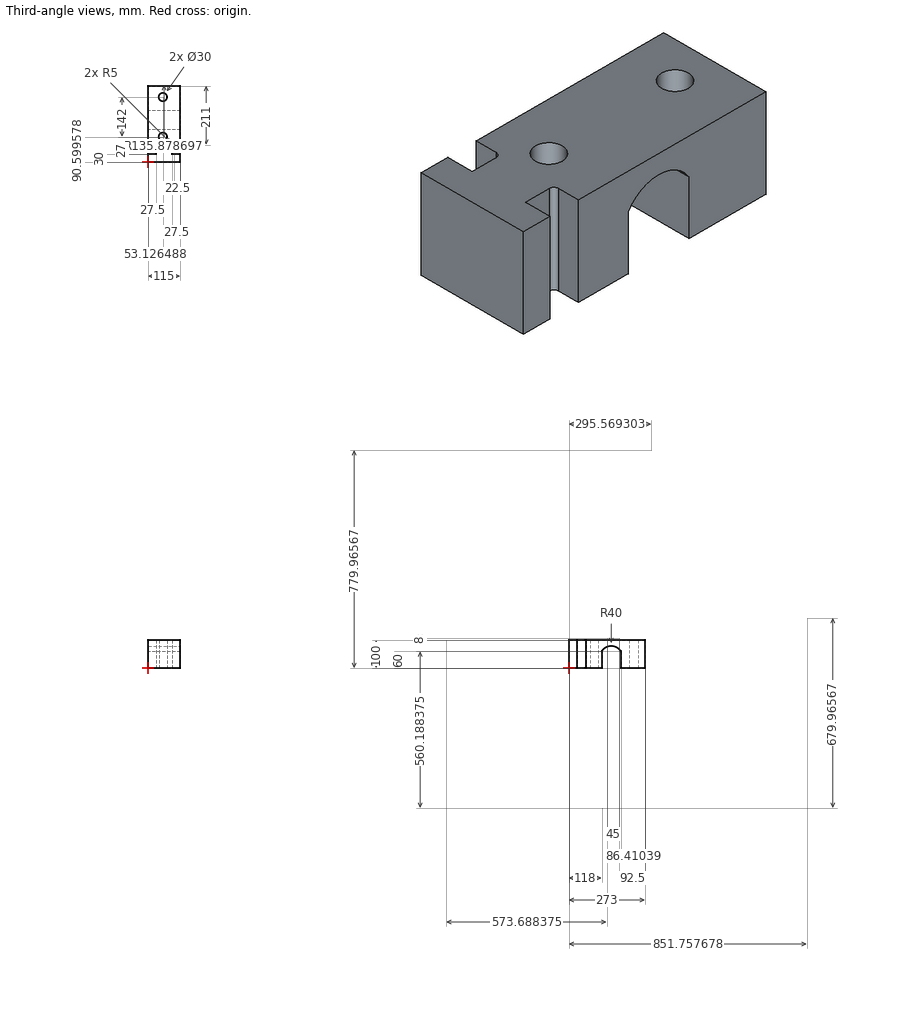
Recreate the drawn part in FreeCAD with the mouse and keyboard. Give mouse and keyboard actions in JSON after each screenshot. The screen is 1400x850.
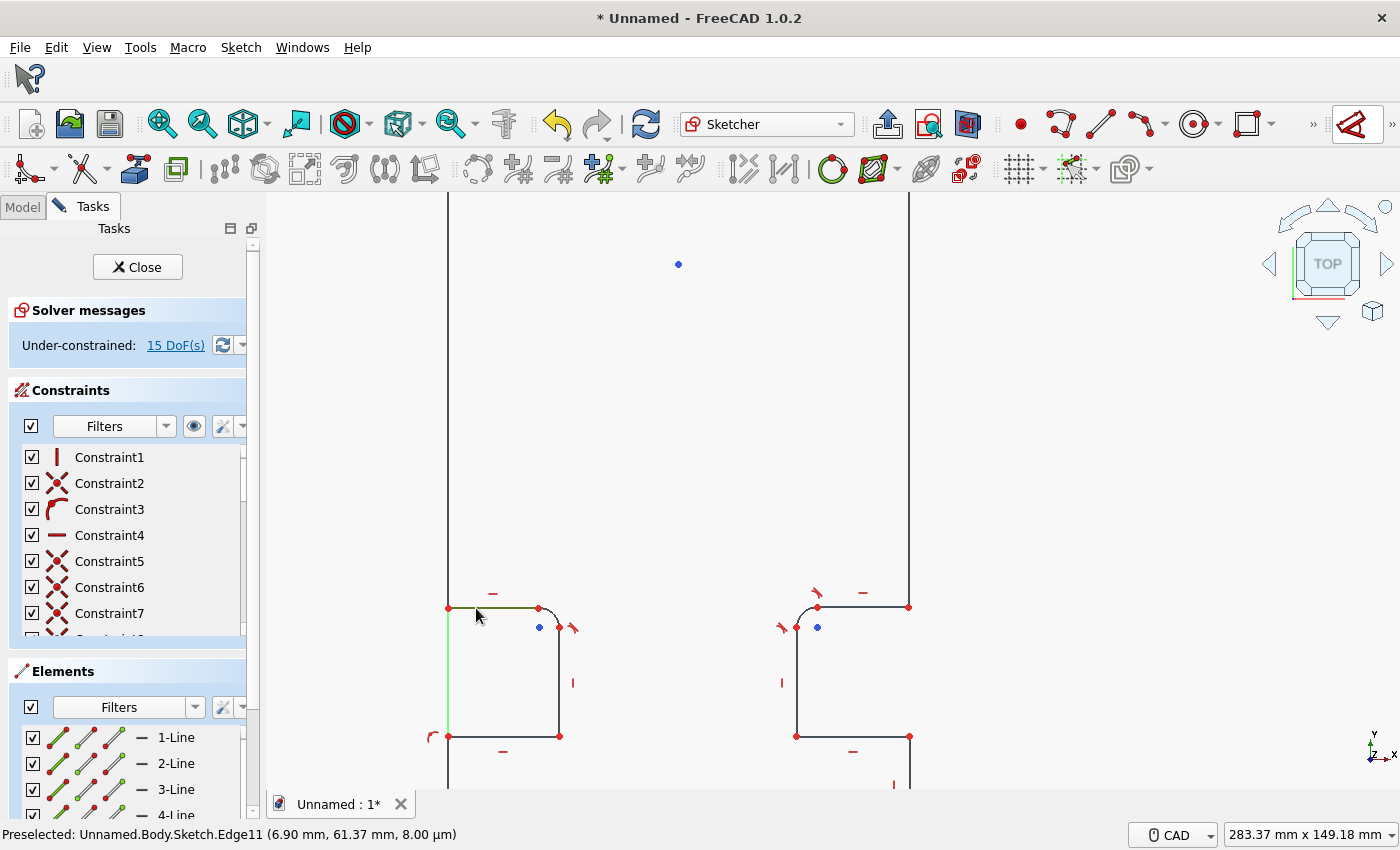
{"action": "scroll", "coordinate": [557, 619], "scroll_direction": "up", "scroll_amount": 2}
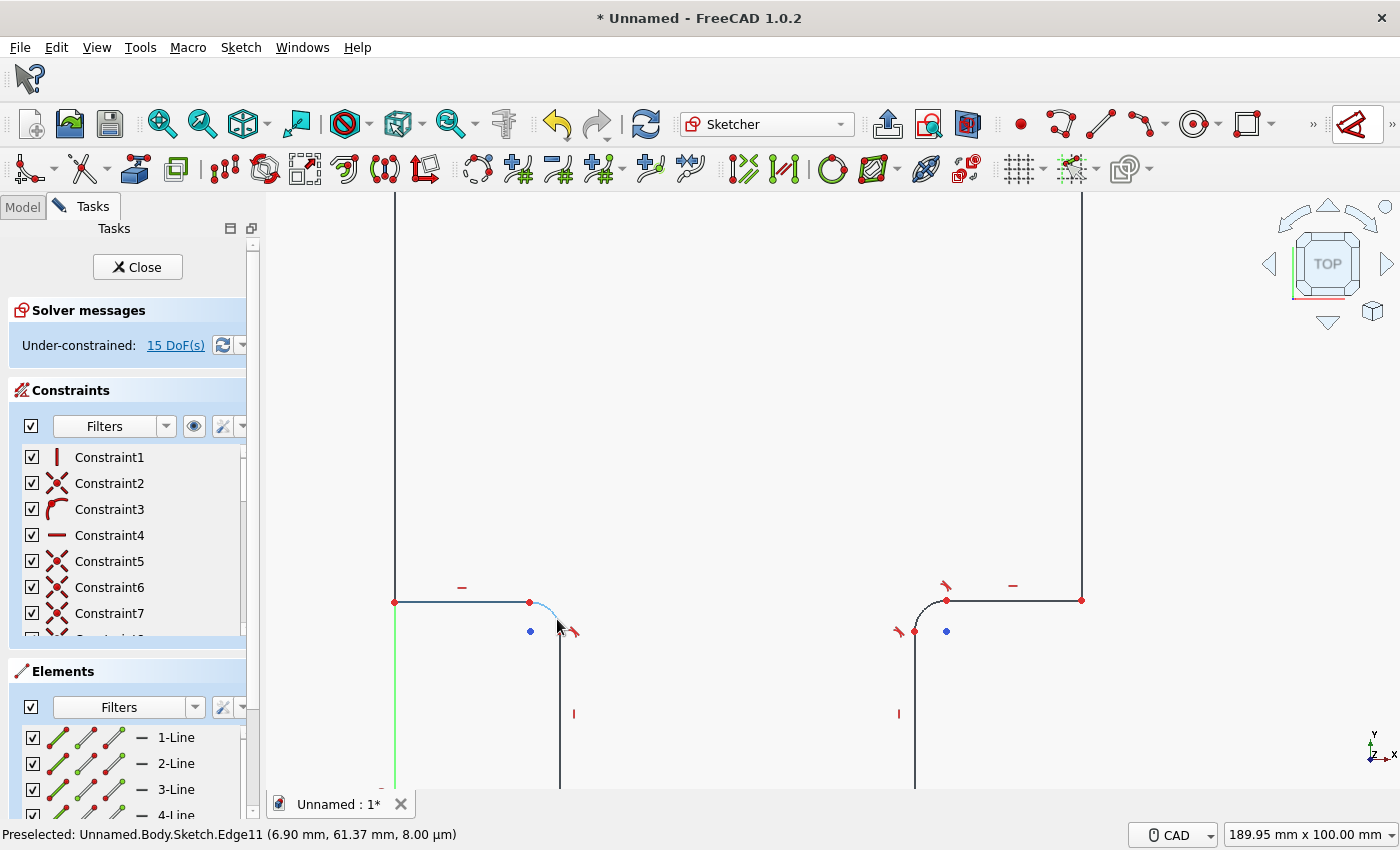
{"action": "left_click", "coordinate": [557, 618]}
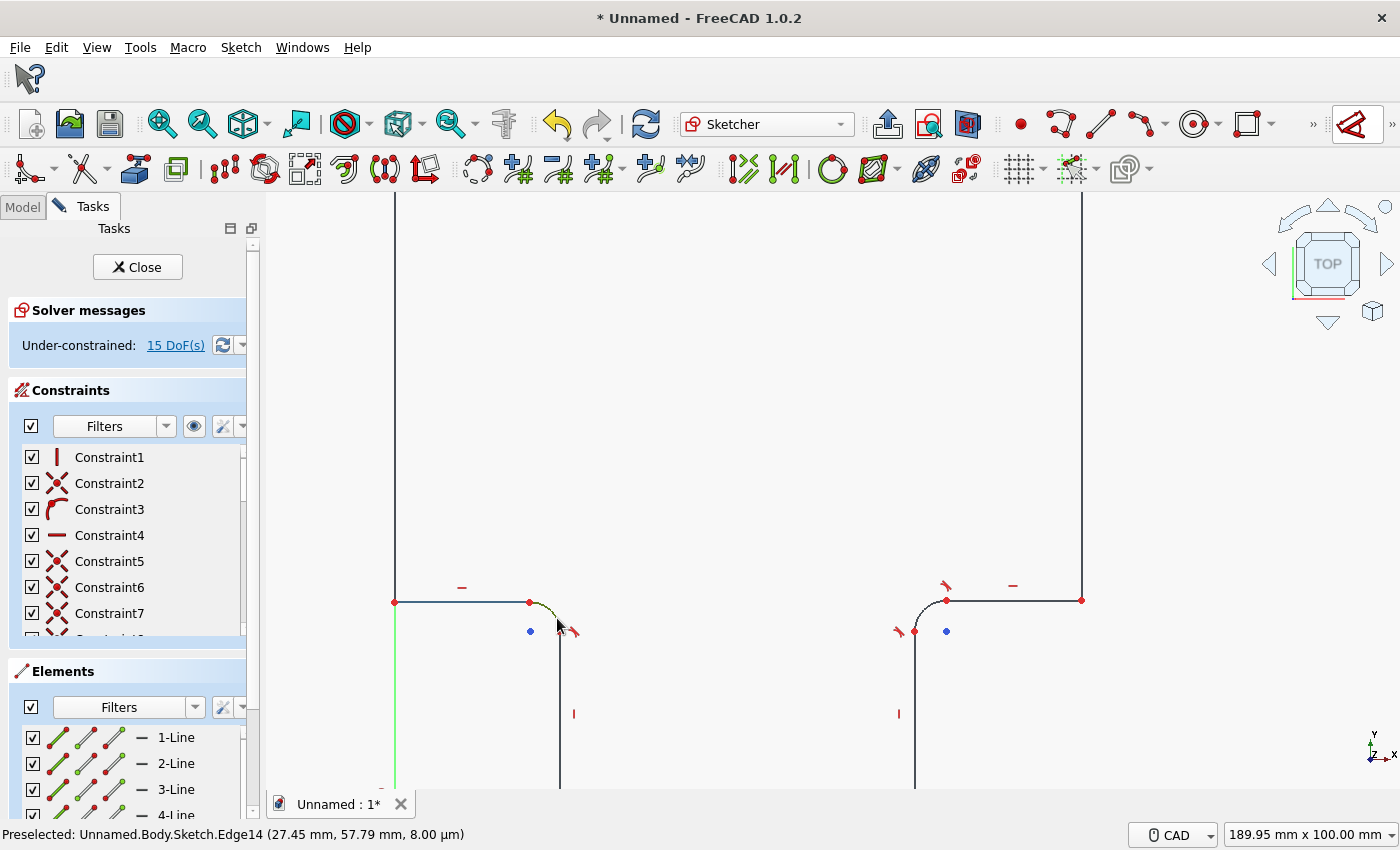
{"action": "key", "text": "t"}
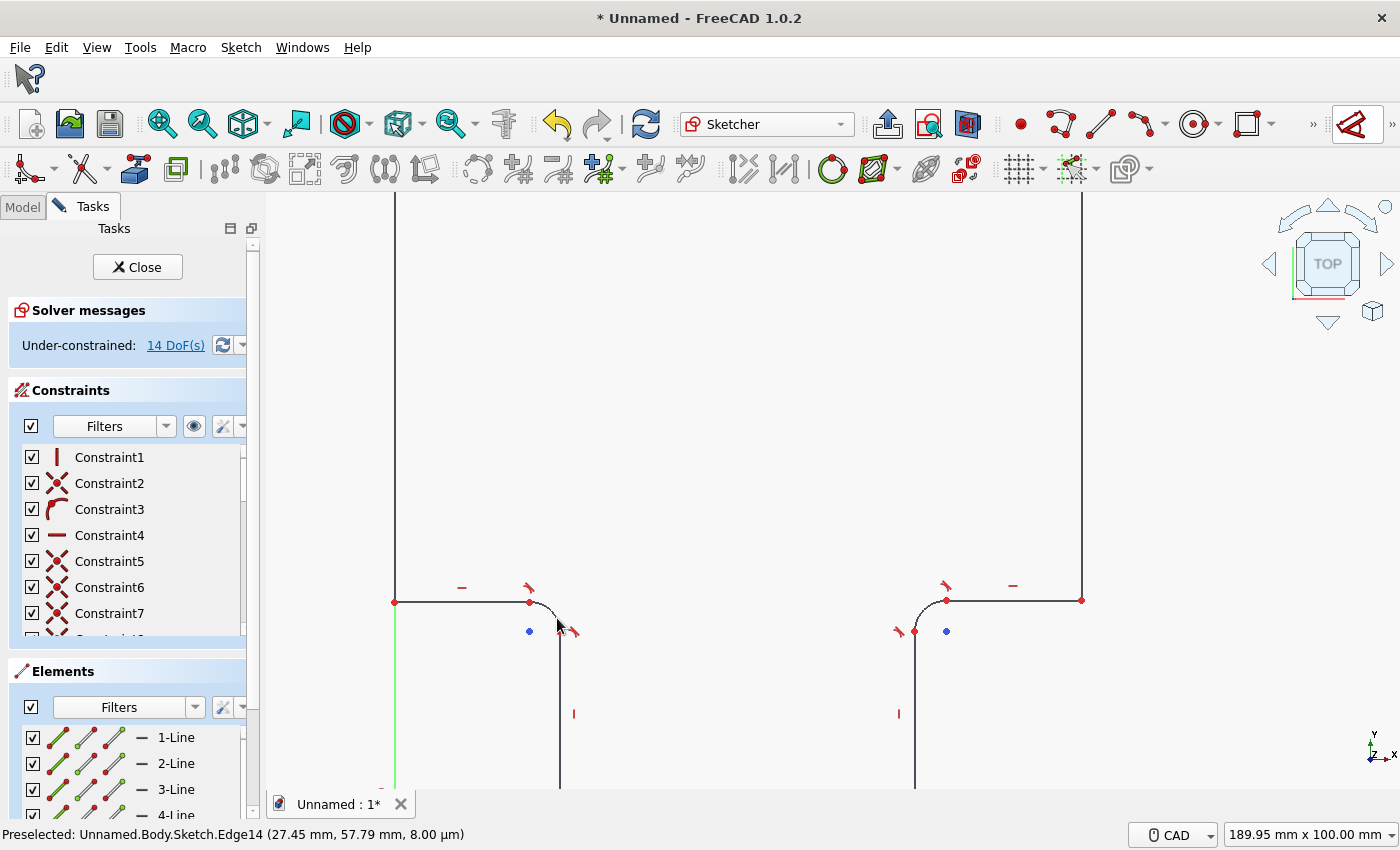
{"action": "scroll", "coordinate": [773, 613], "scroll_direction": "down", "scroll_amount": 7}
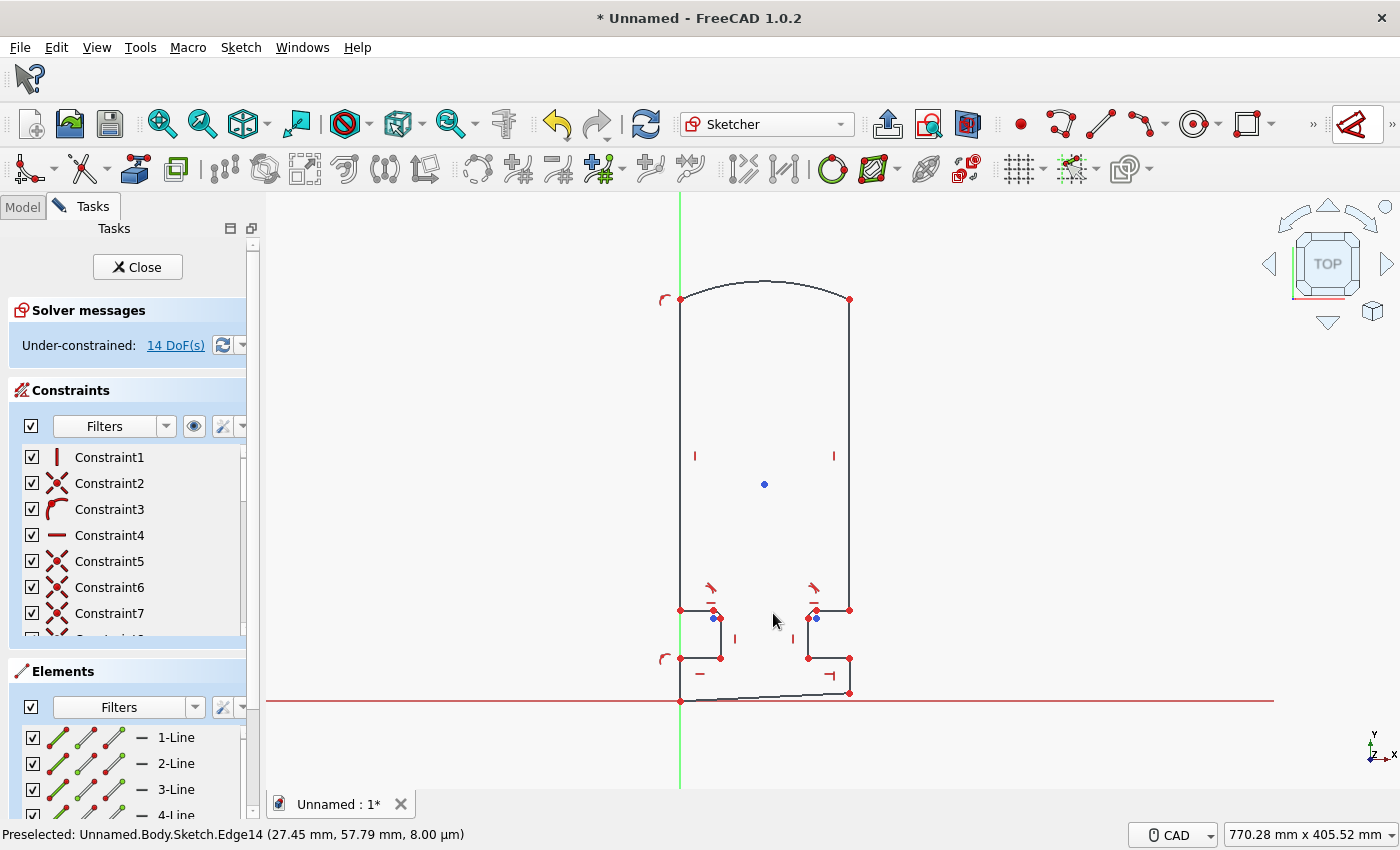
{"action": "scroll", "coordinate": [731, 699], "scroll_direction": "up", "scroll_amount": 9}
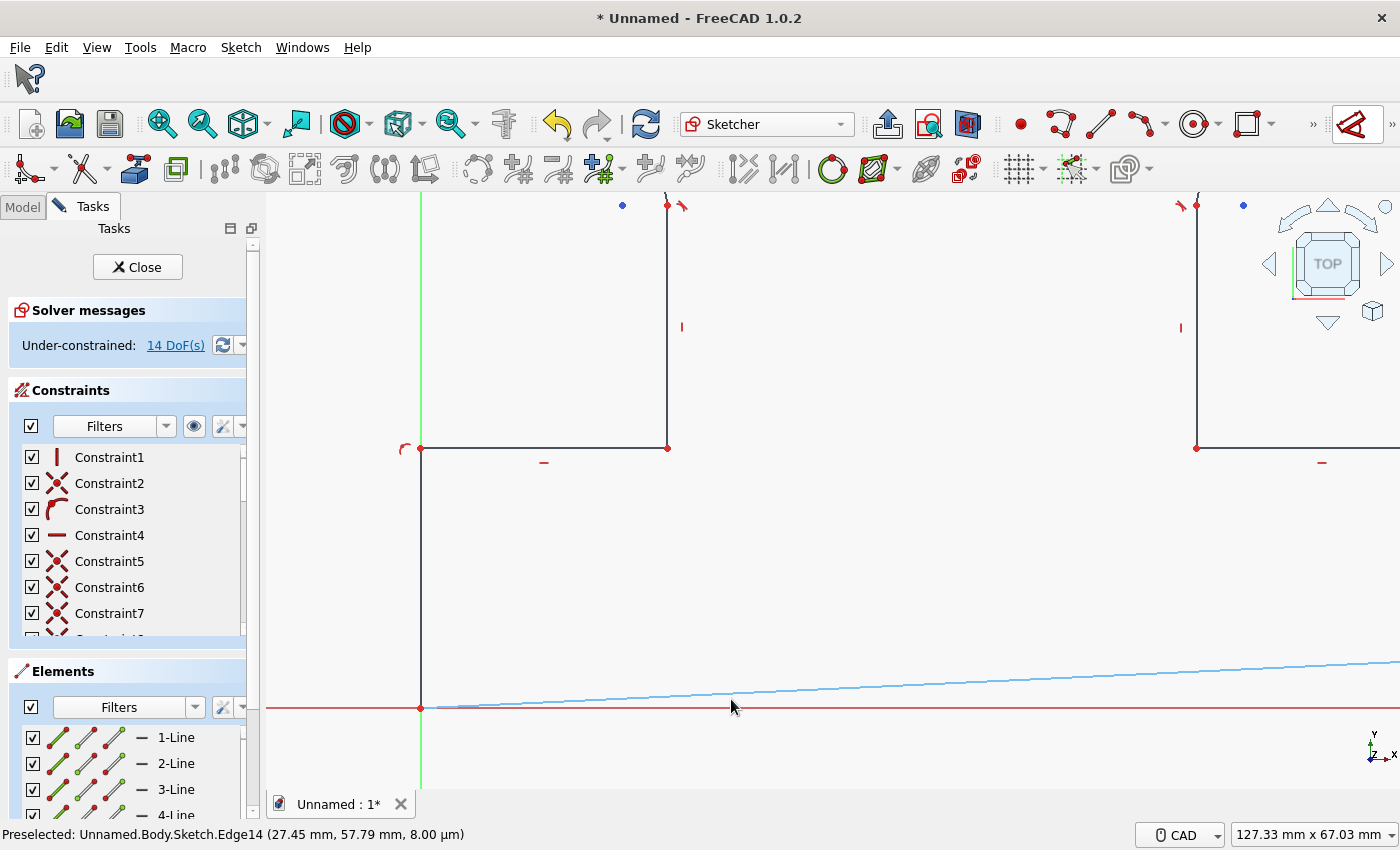
{"action": "left_click", "coordinate": [729, 694]}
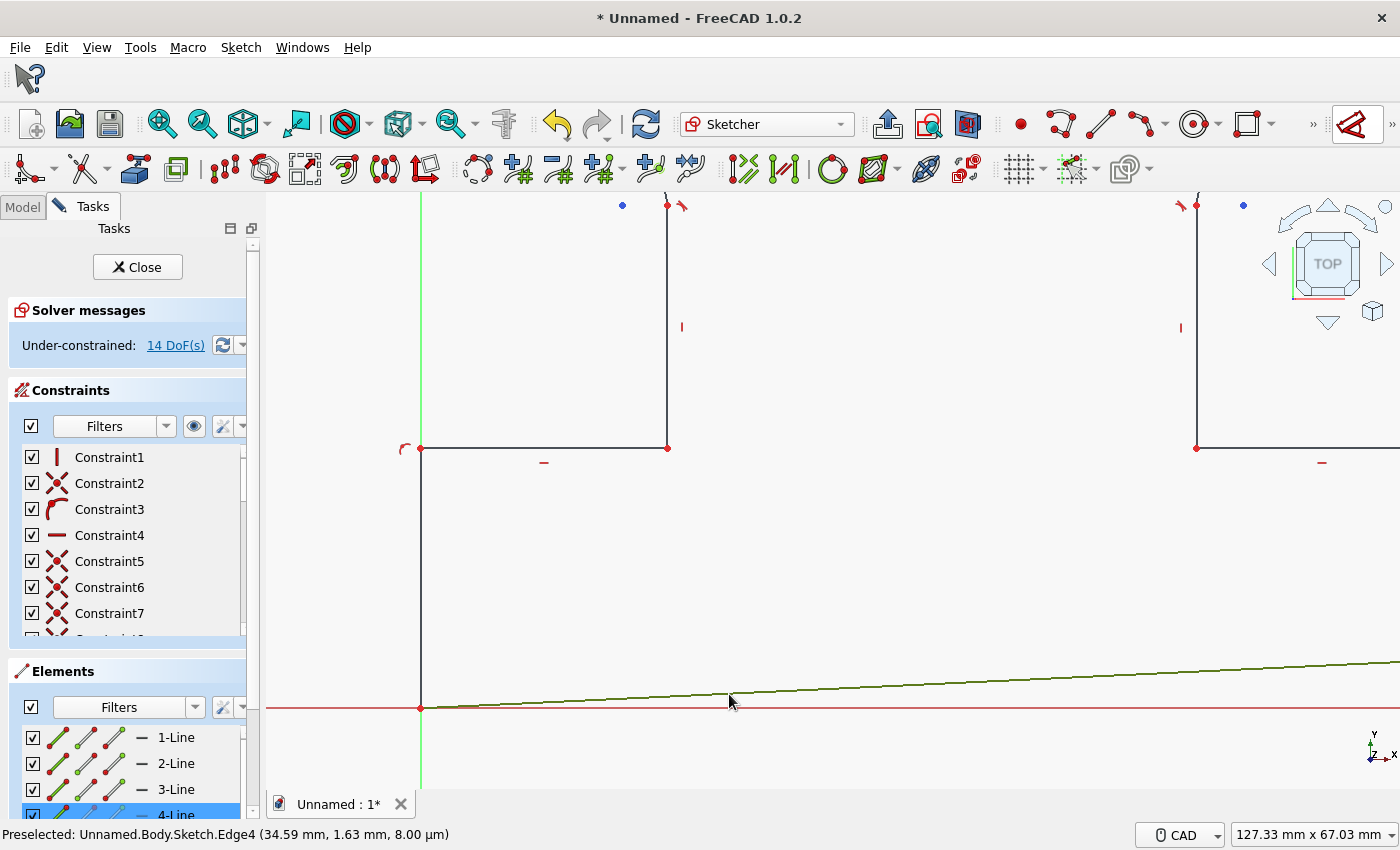
{"action": "key", "text": "h"}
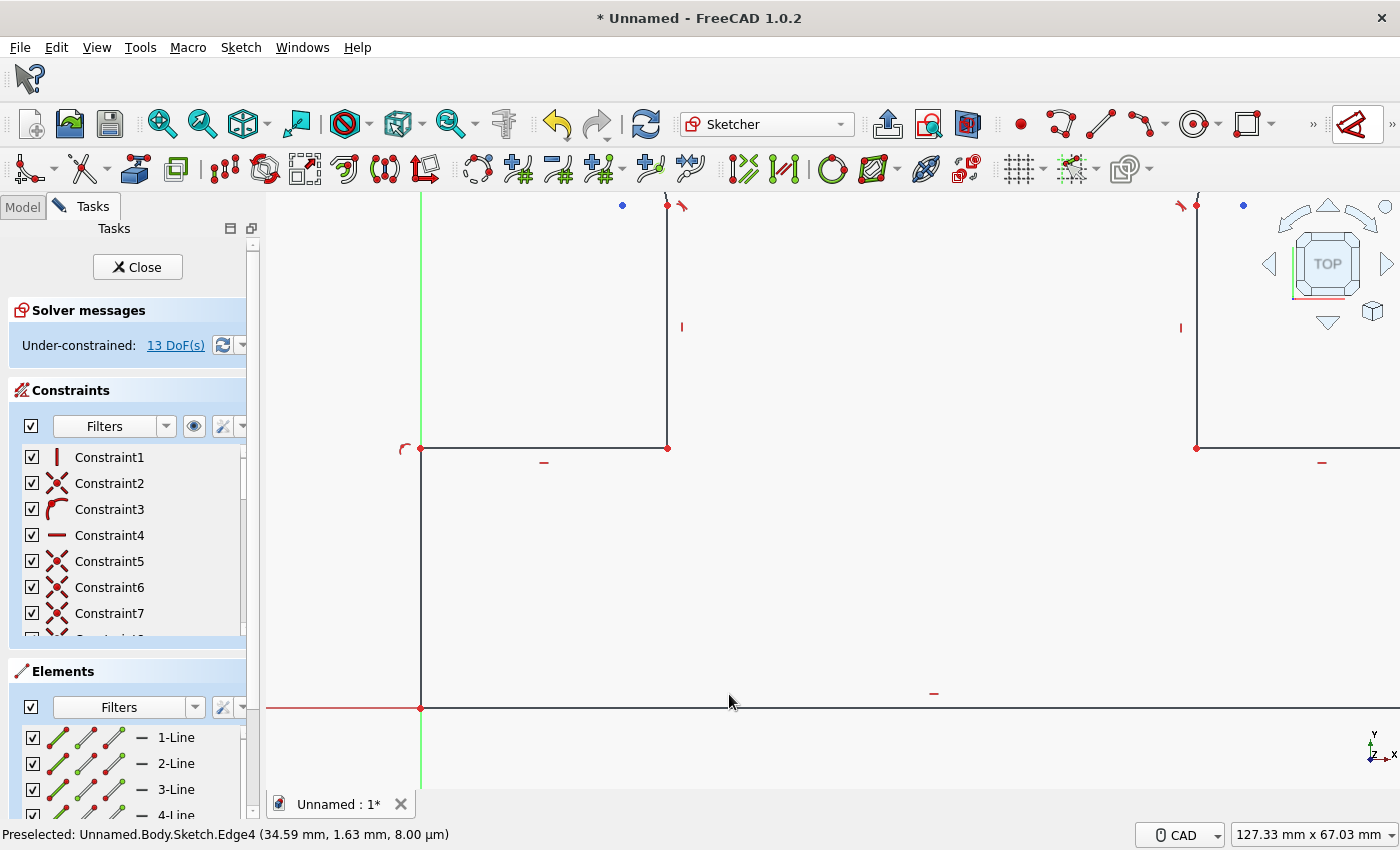
{"action": "scroll", "coordinate": [731, 699], "scroll_direction": "down", "scroll_amount": 9}